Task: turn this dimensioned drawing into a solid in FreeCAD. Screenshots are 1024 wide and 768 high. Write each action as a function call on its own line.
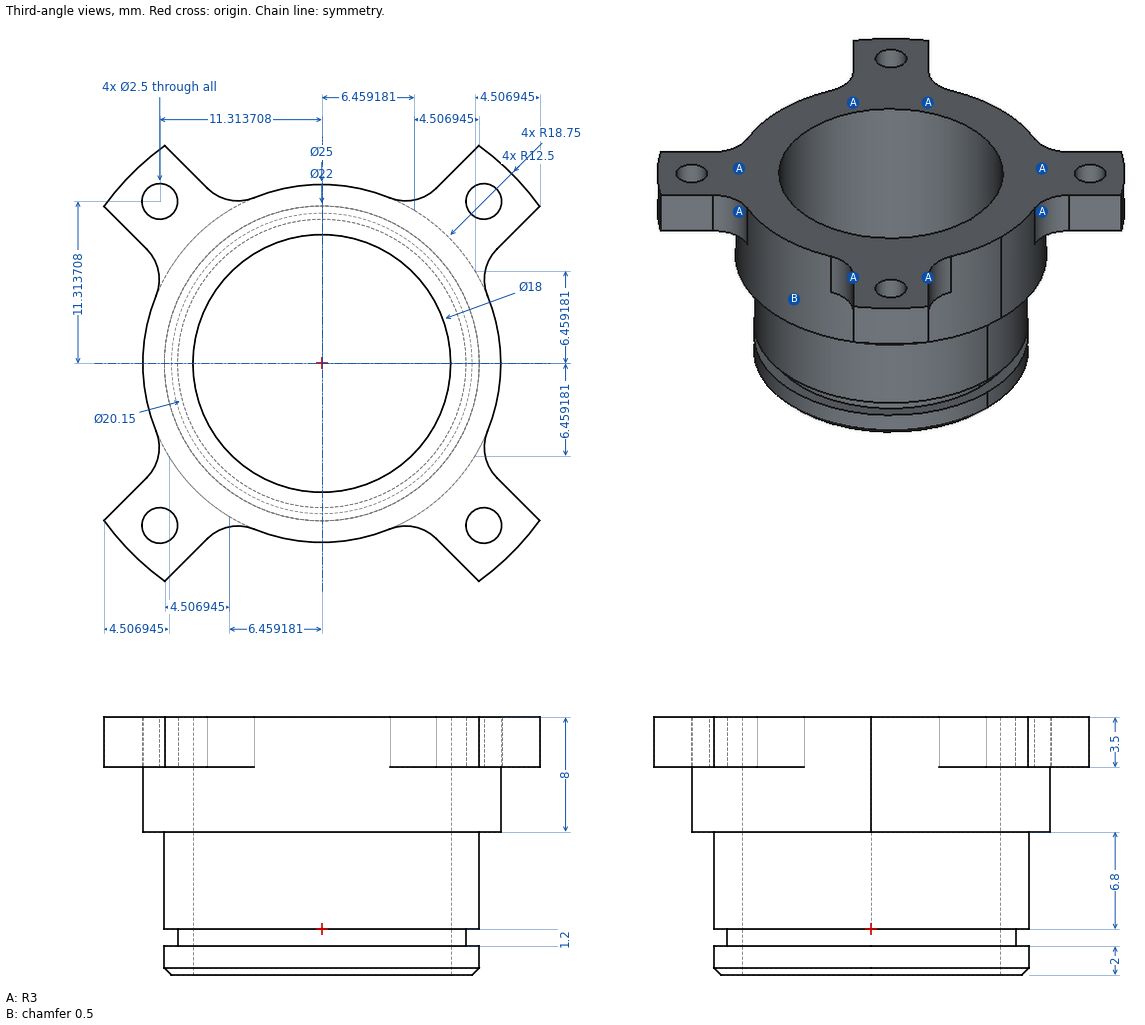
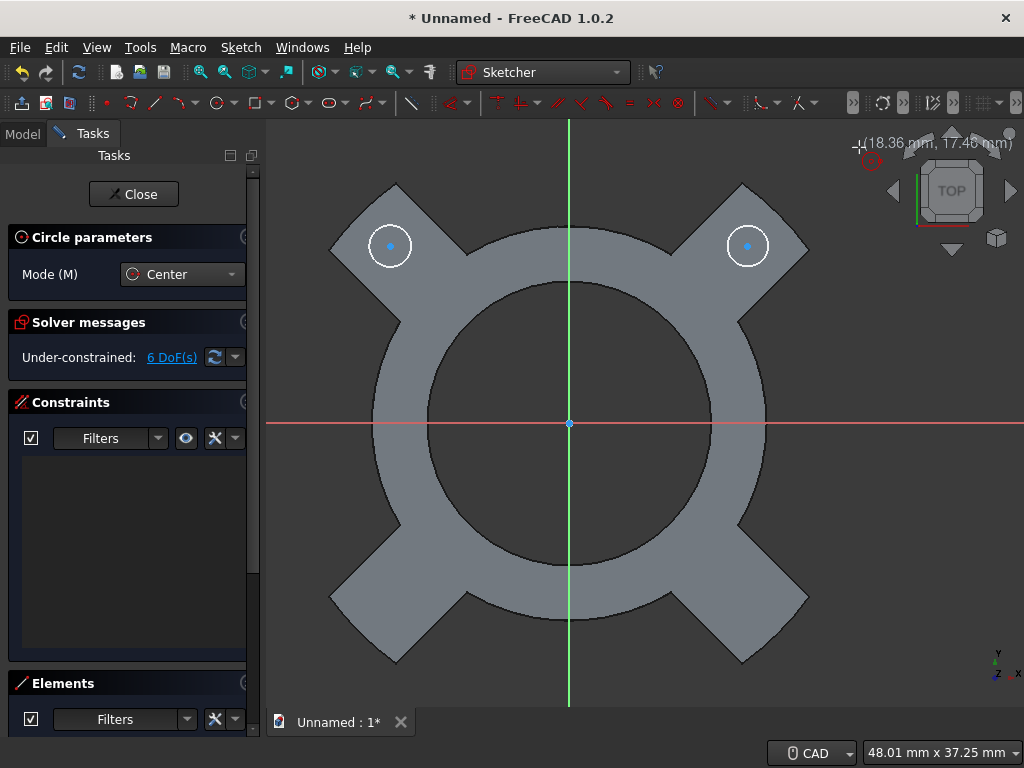
click(748, 602)
click(762, 588)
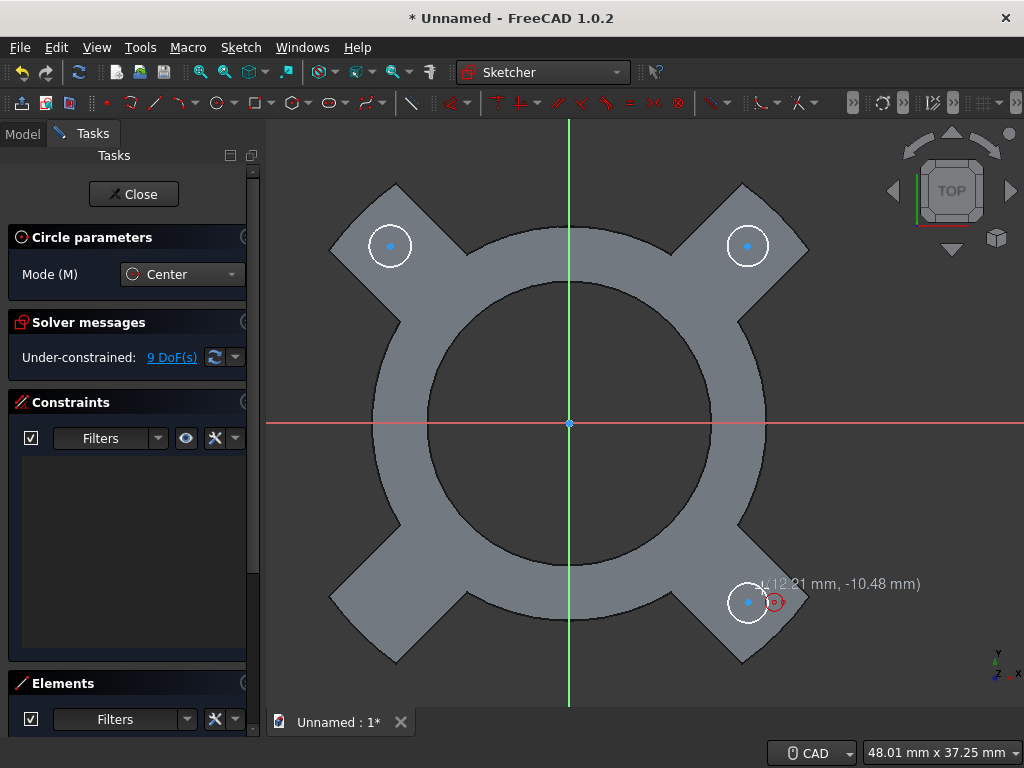
click(391, 602)
click(405, 588)
key(Escape)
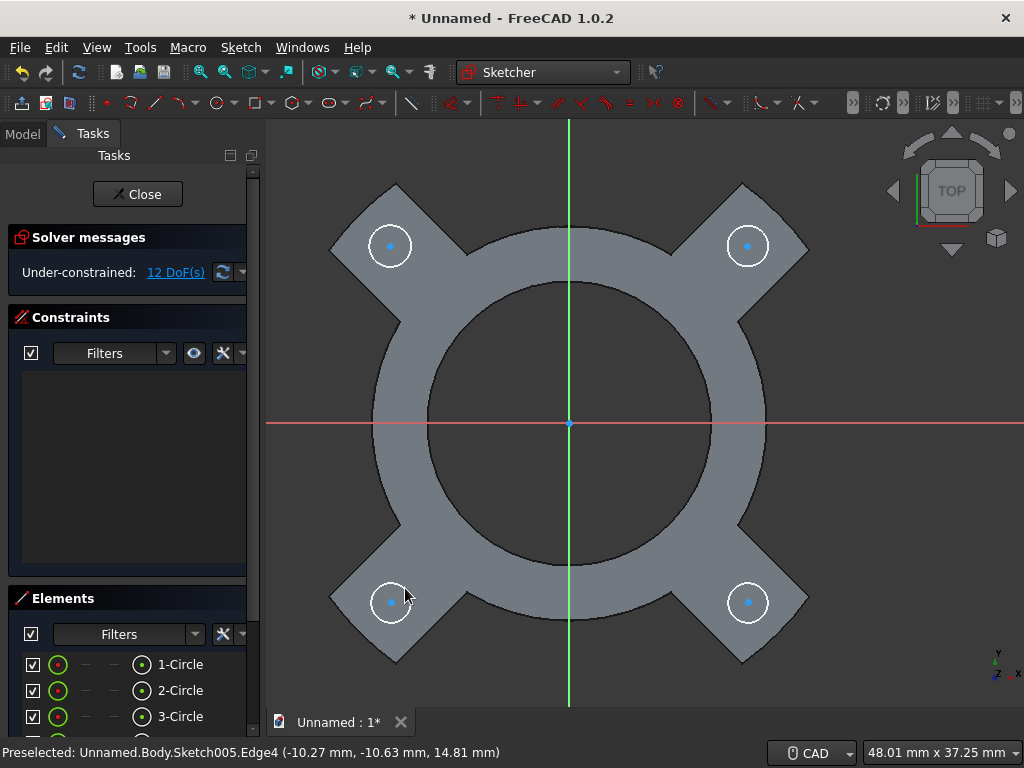
click(405, 231)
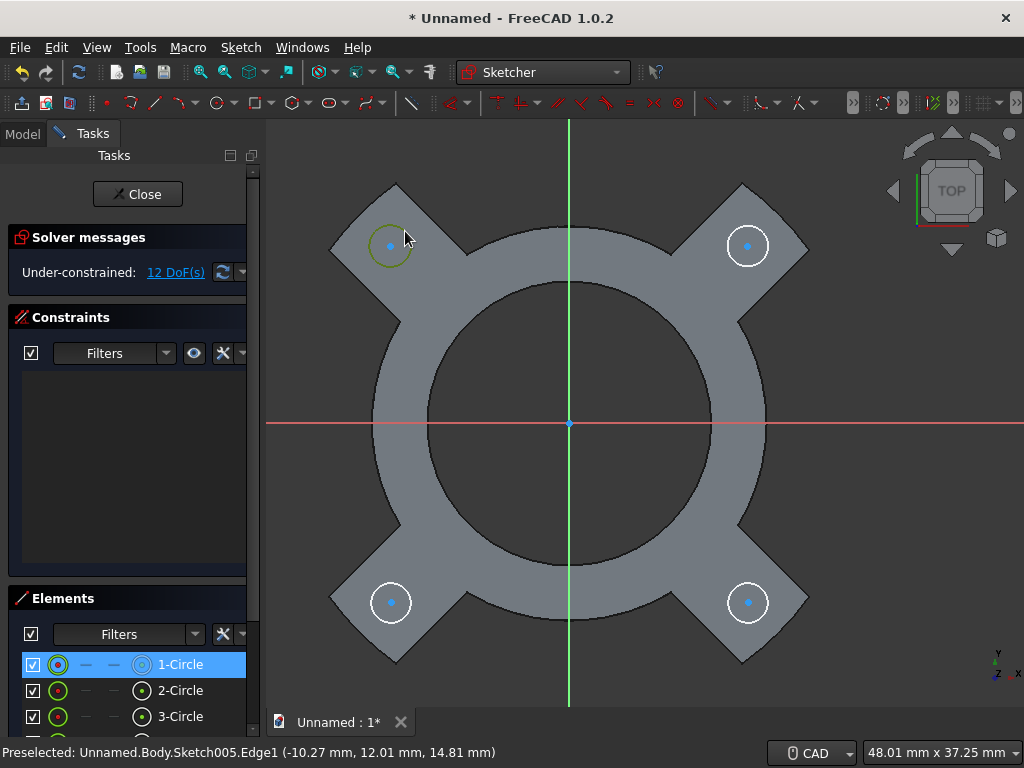
click(762, 232)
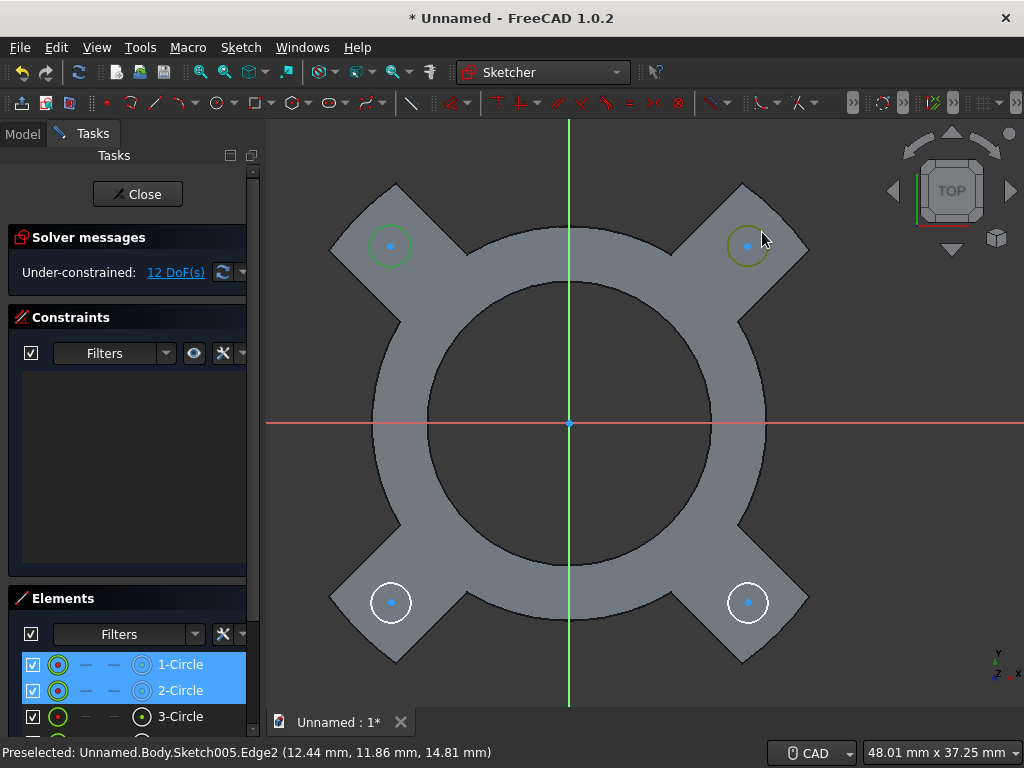
click(762, 589)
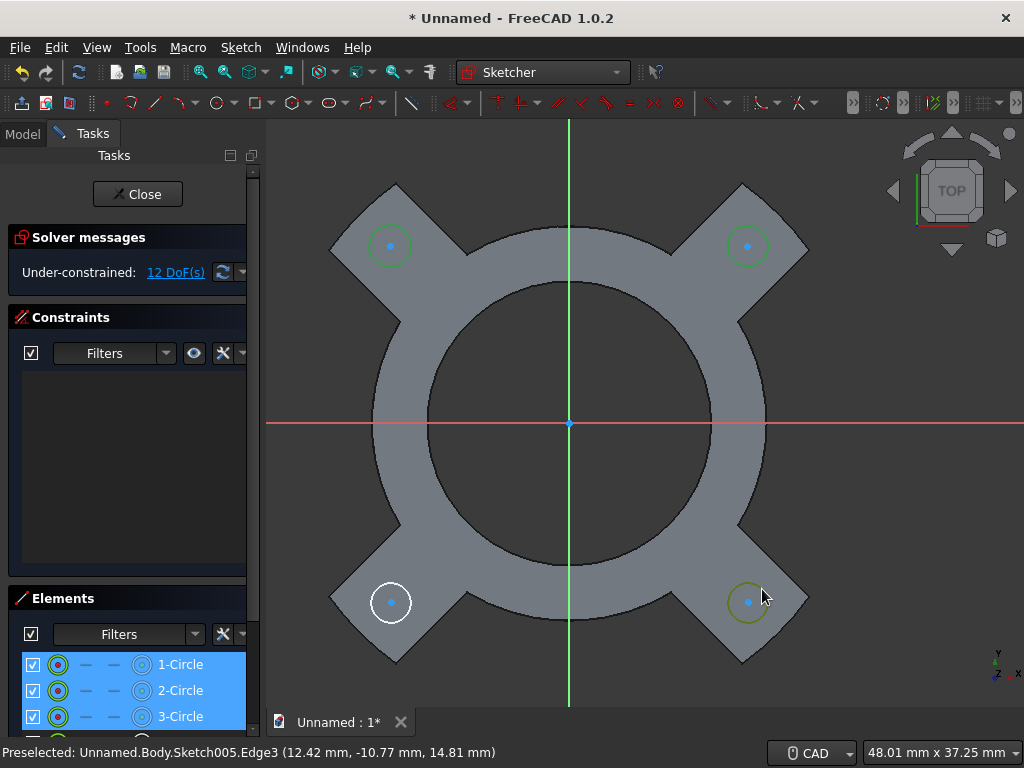
click(405, 589)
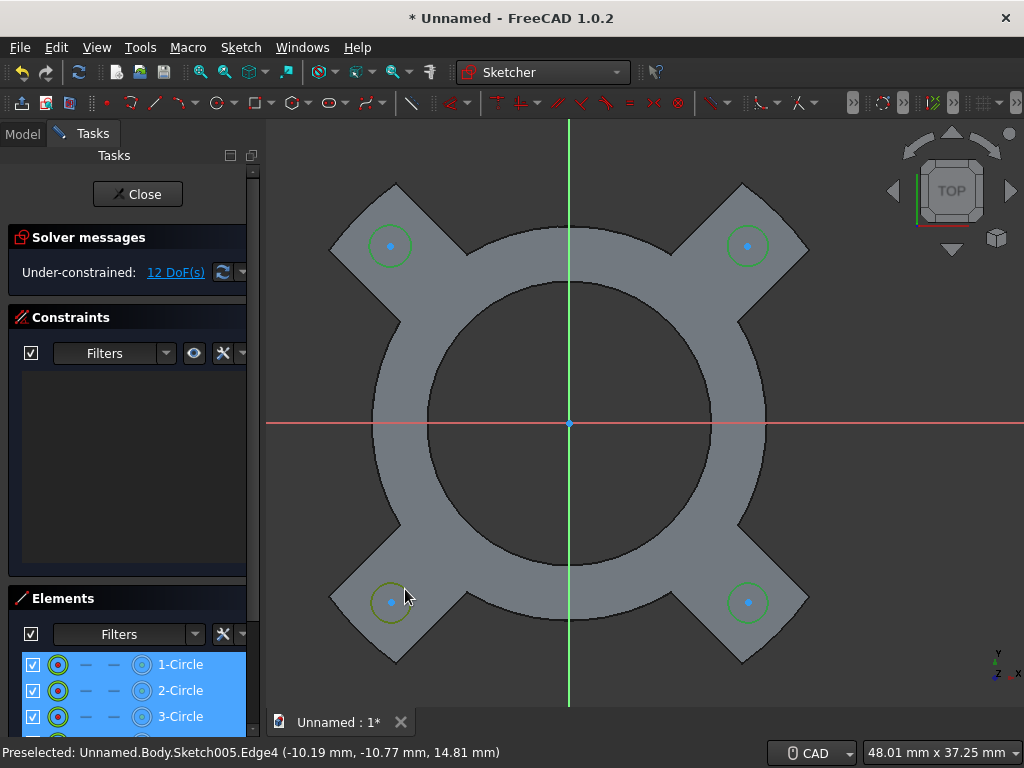
click(630, 104)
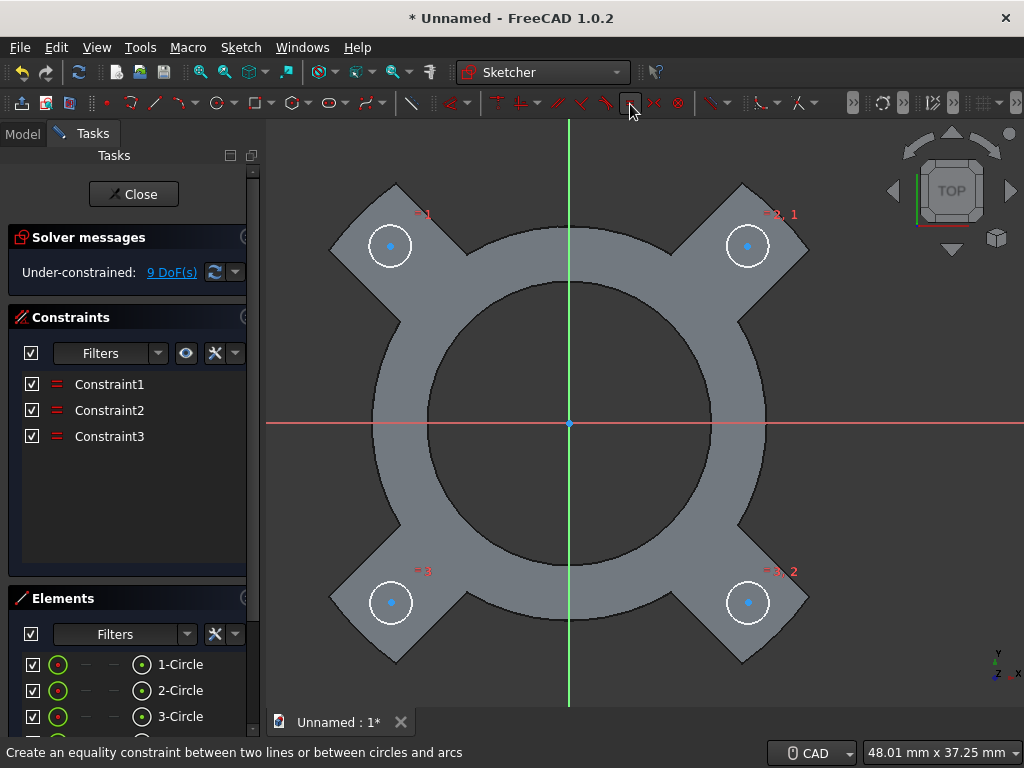
click(390, 246)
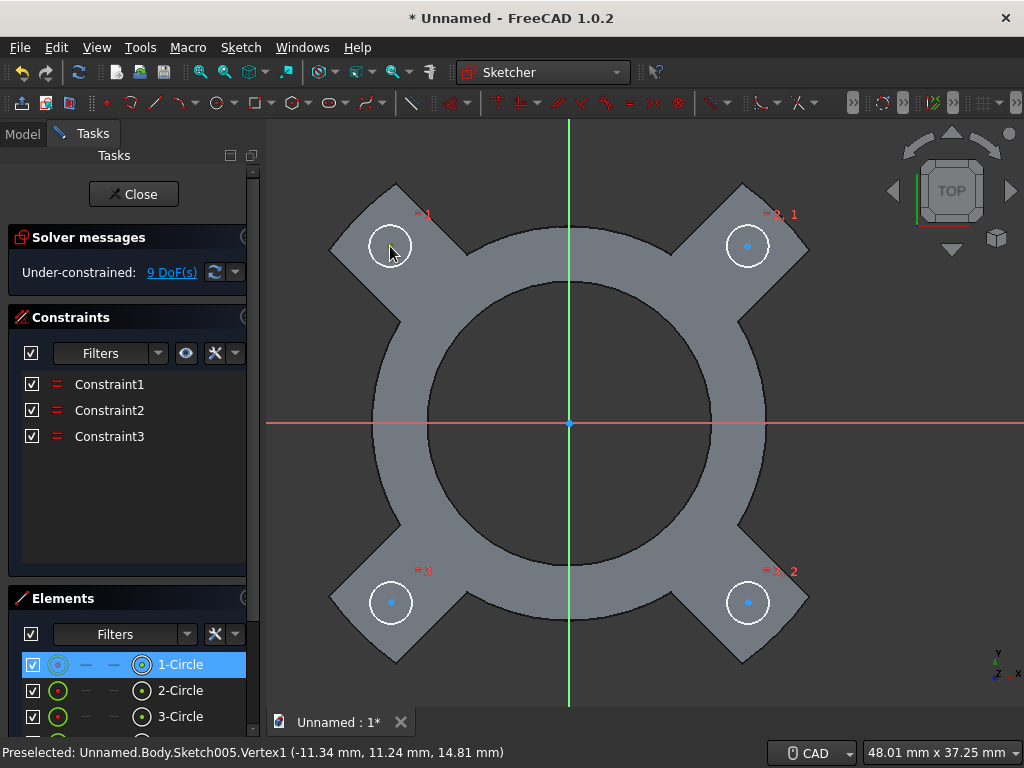
click(748, 246)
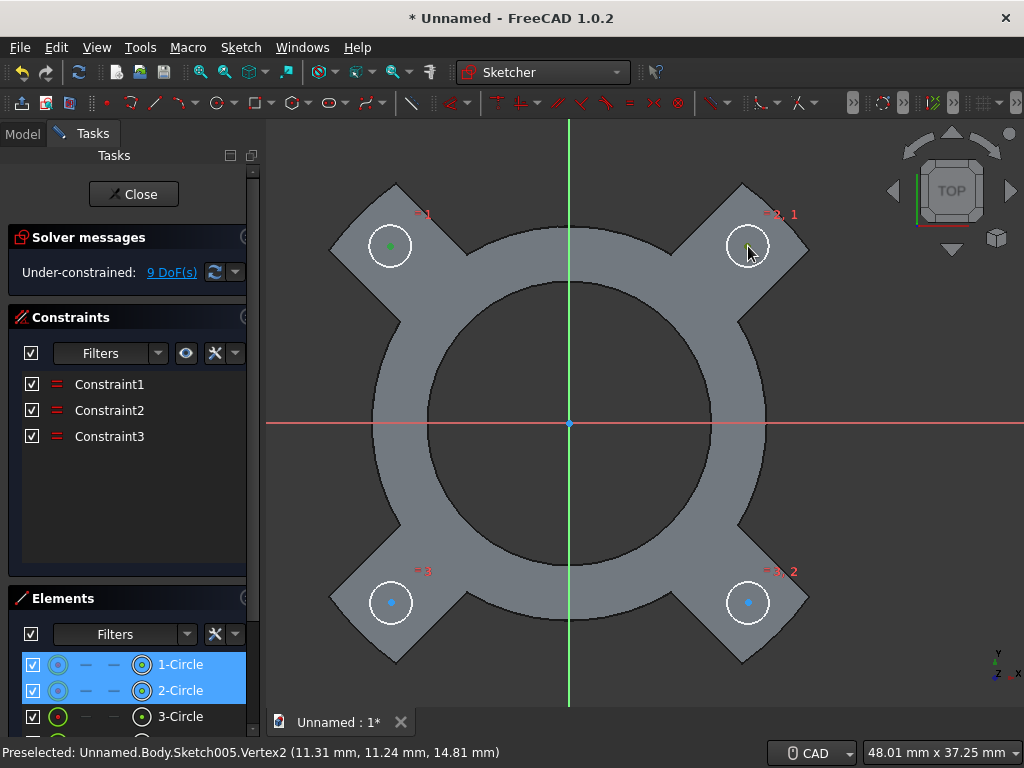
click(569, 641)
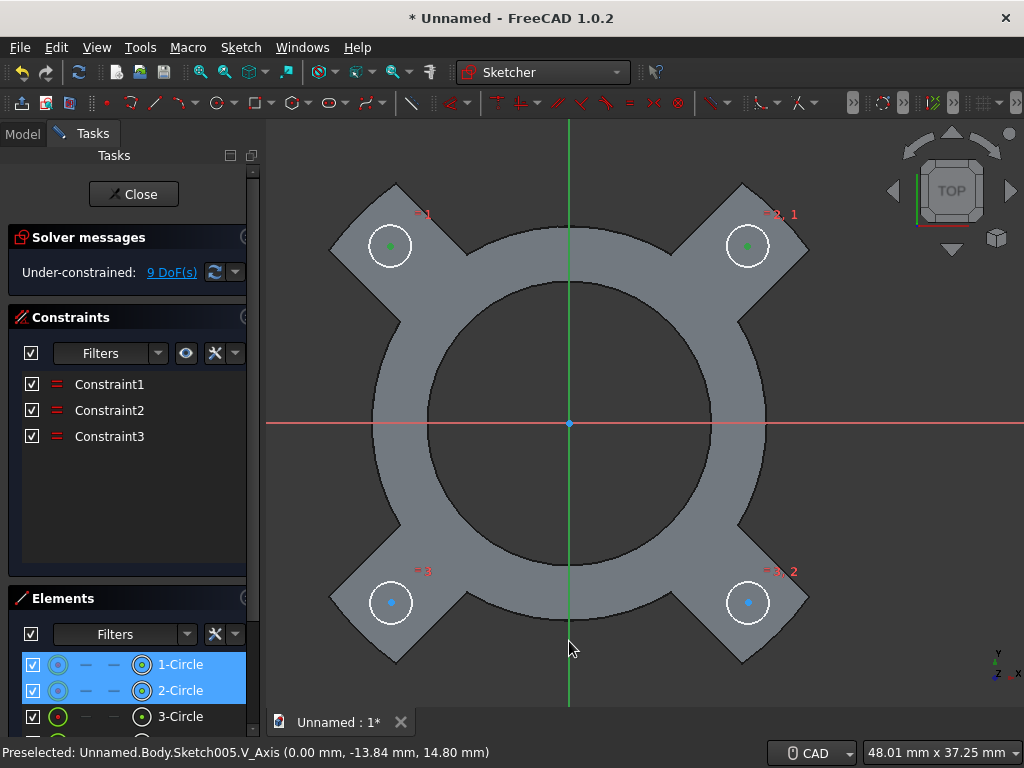
click(654, 104)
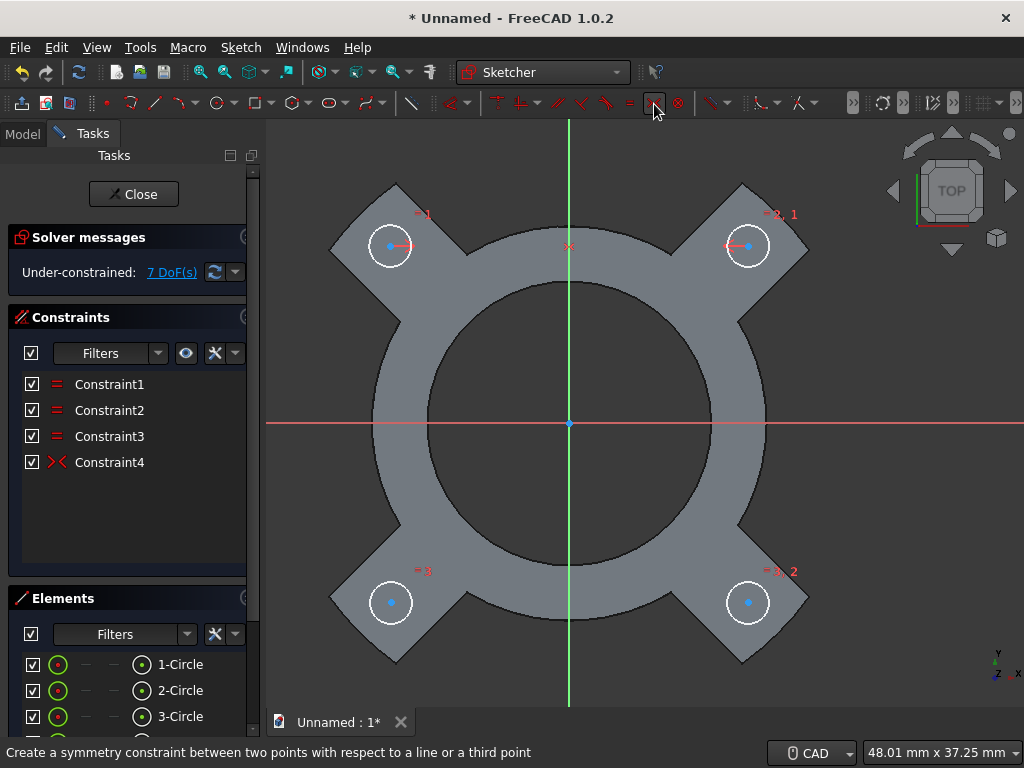
click(748, 246)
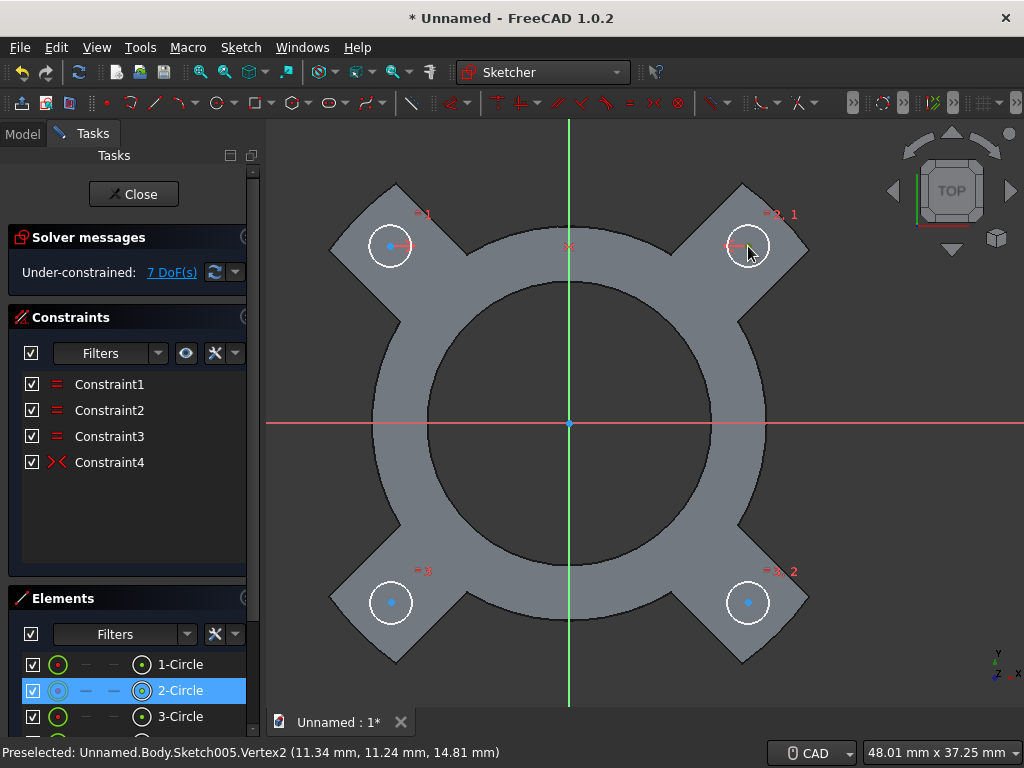
click(748, 603)